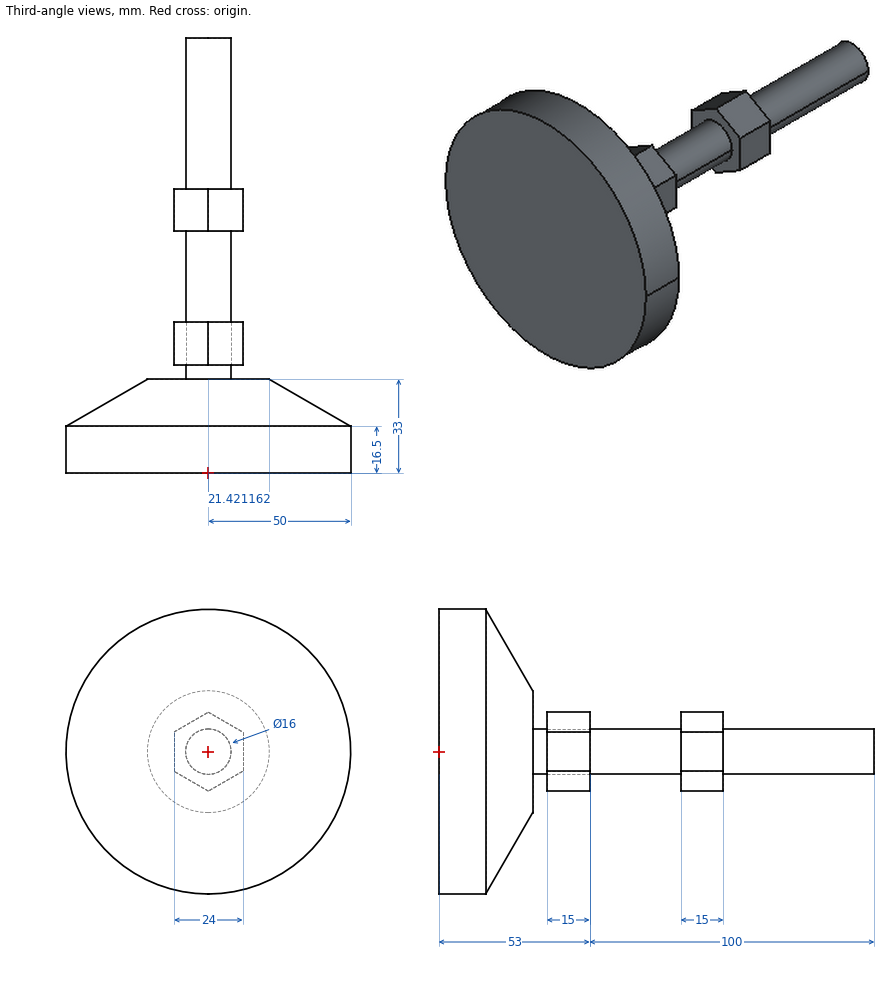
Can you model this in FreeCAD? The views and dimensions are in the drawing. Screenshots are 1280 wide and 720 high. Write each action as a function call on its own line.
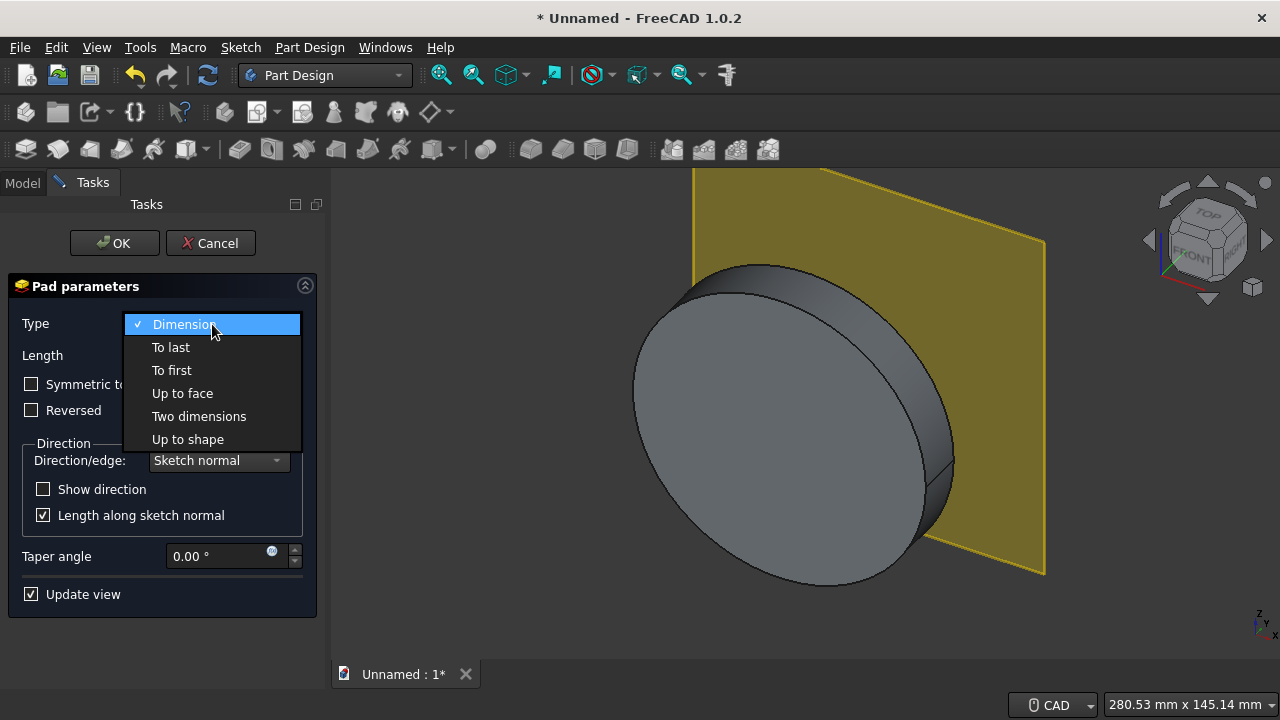
click(212, 416)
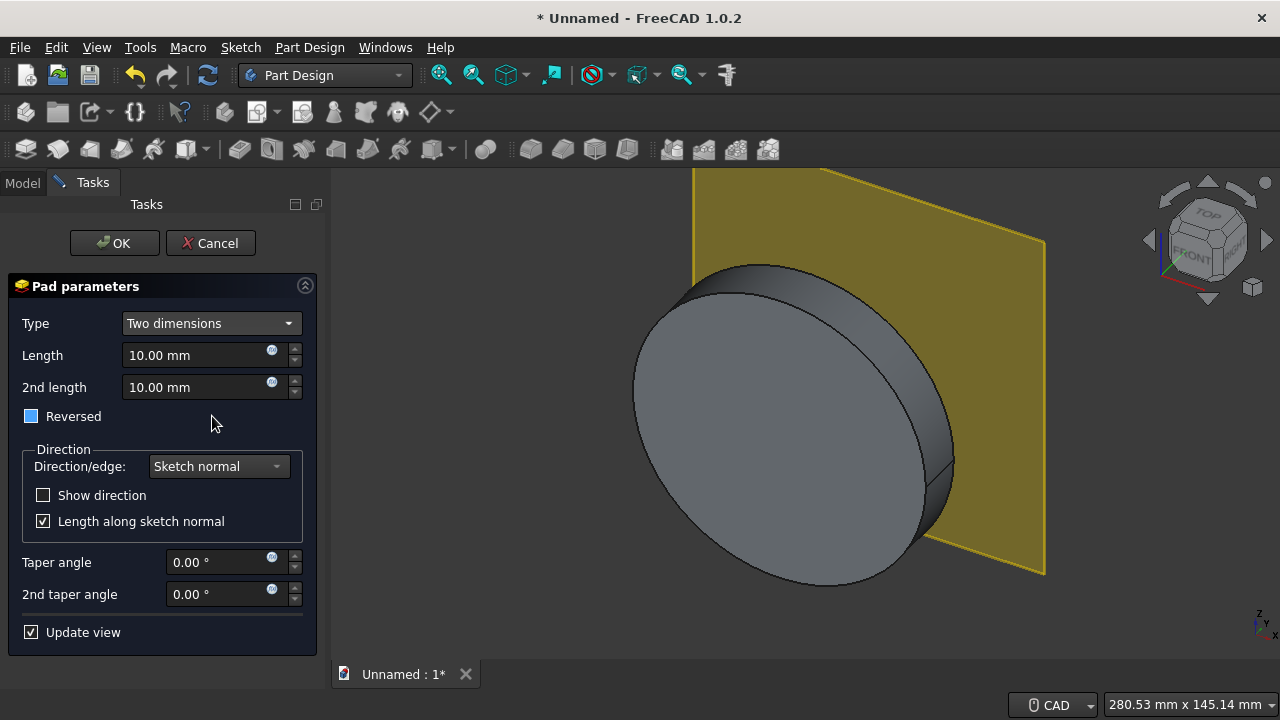
triple_click(204, 355)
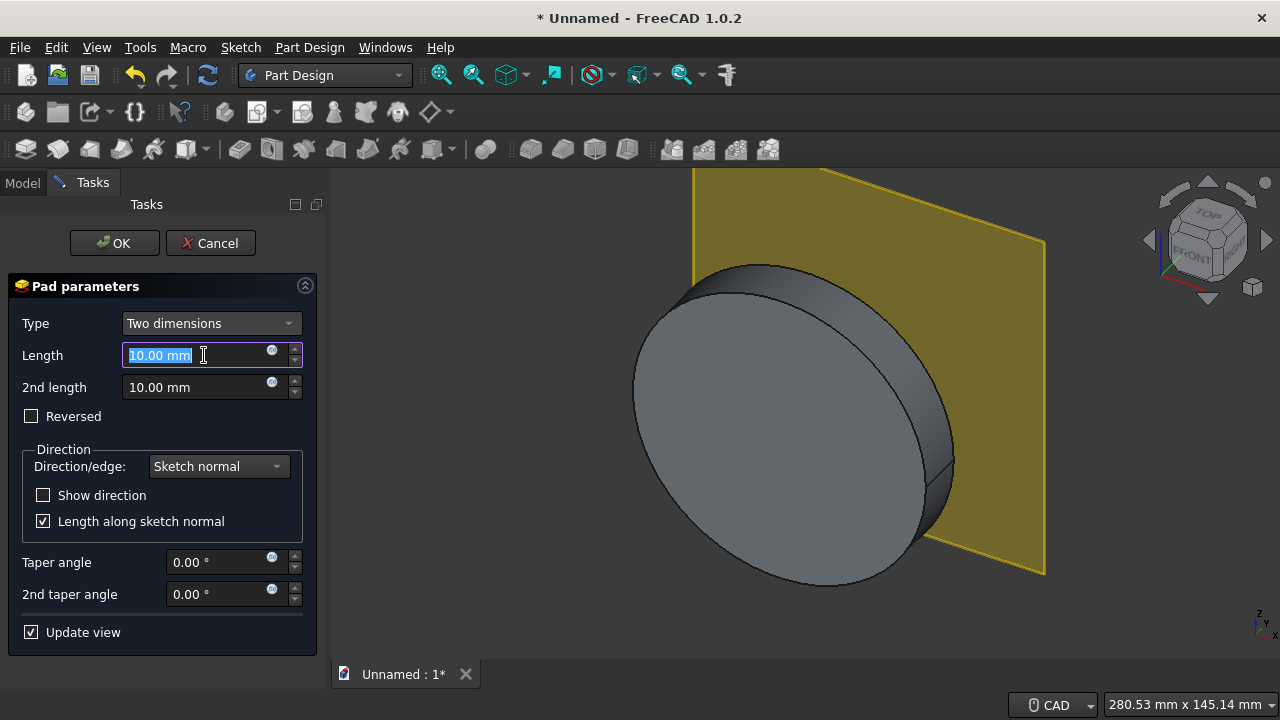
text(100)
key(Tab)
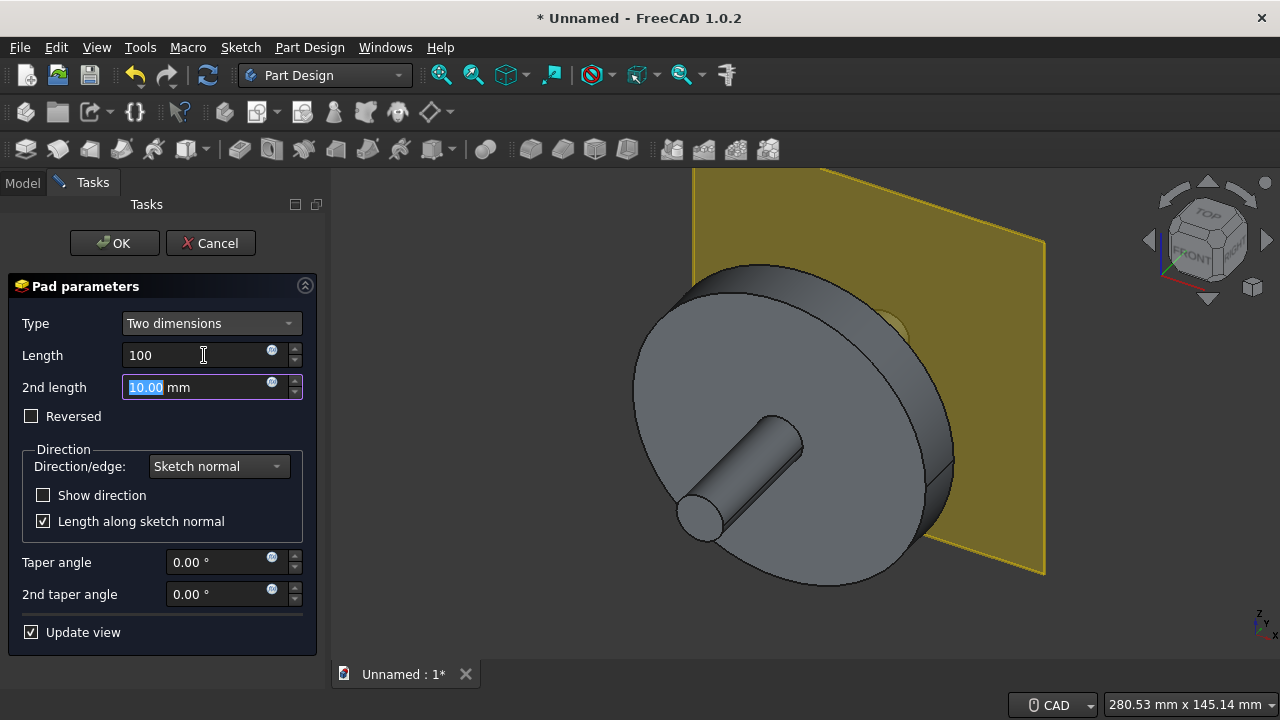
text(53)
key(Tab)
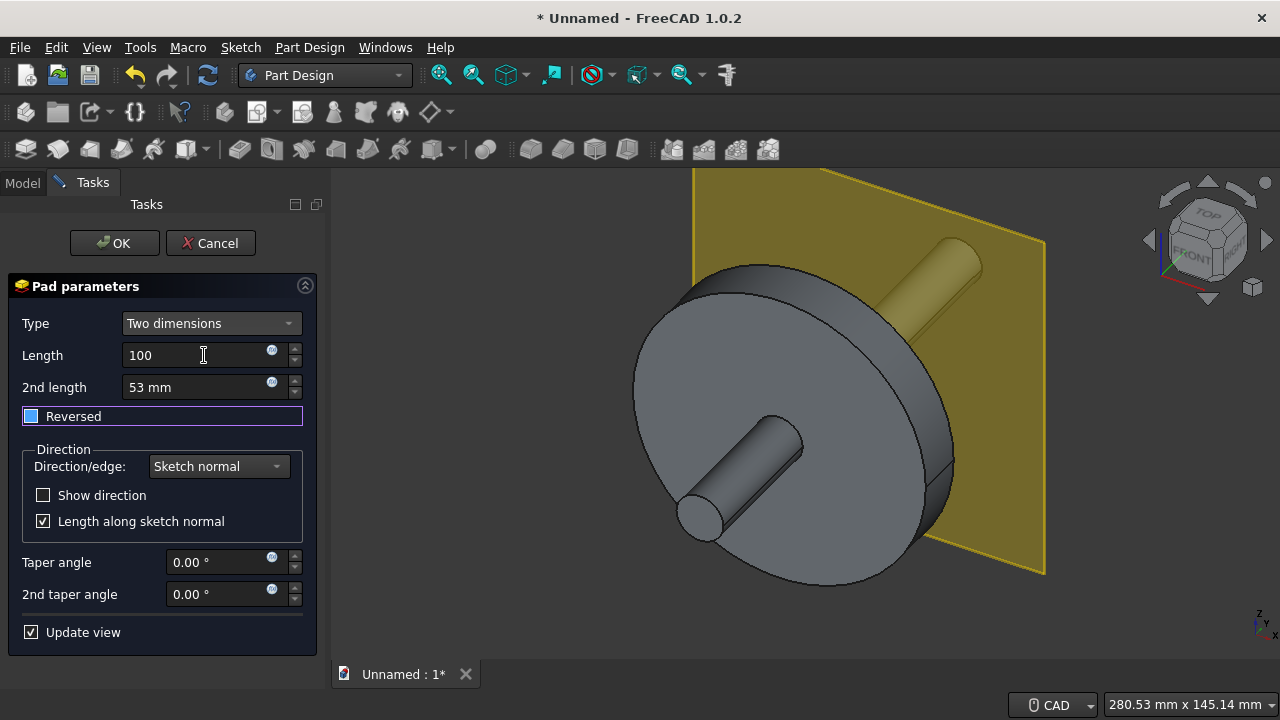
click(30, 416)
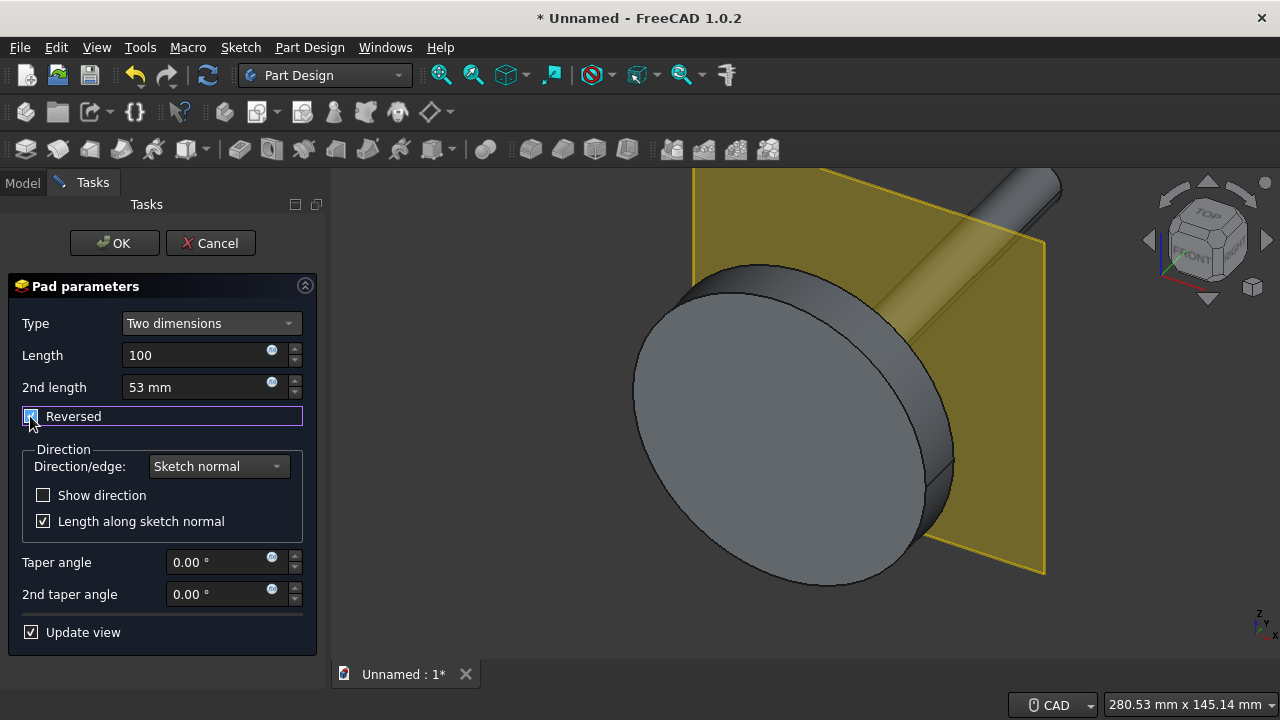
click(115, 243)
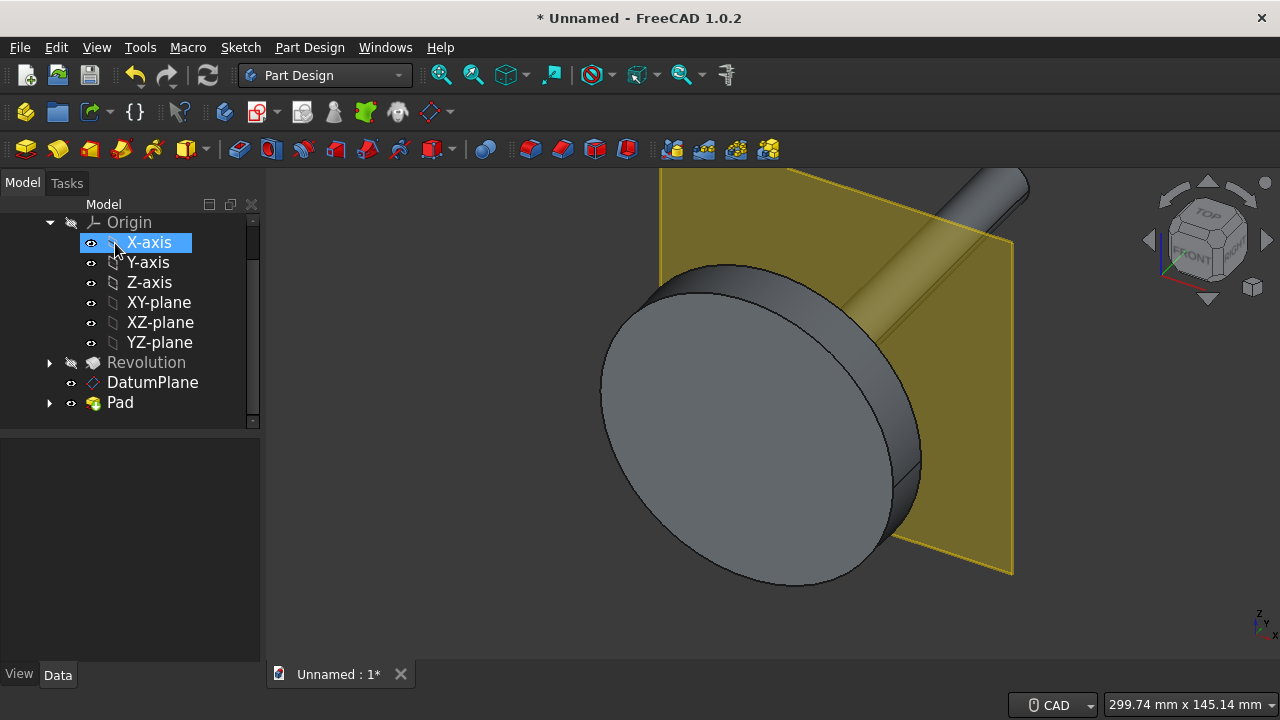
click(116, 383)
key(space)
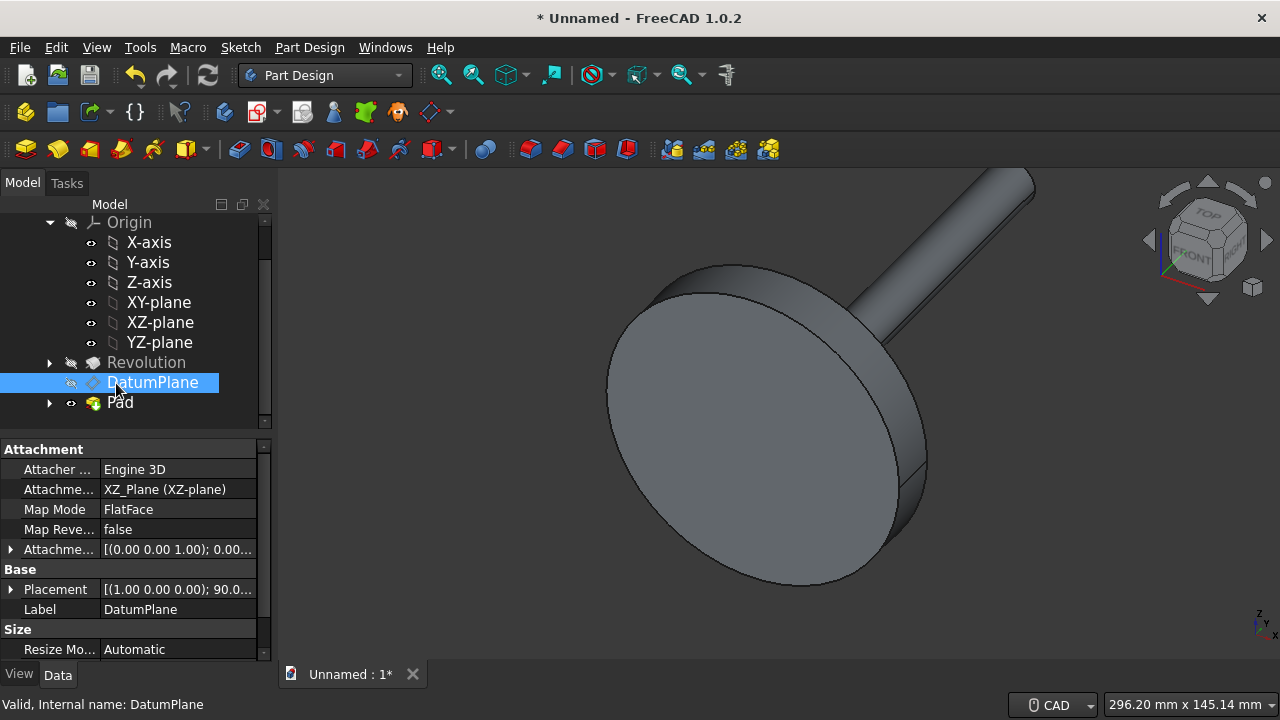
click(442, 76)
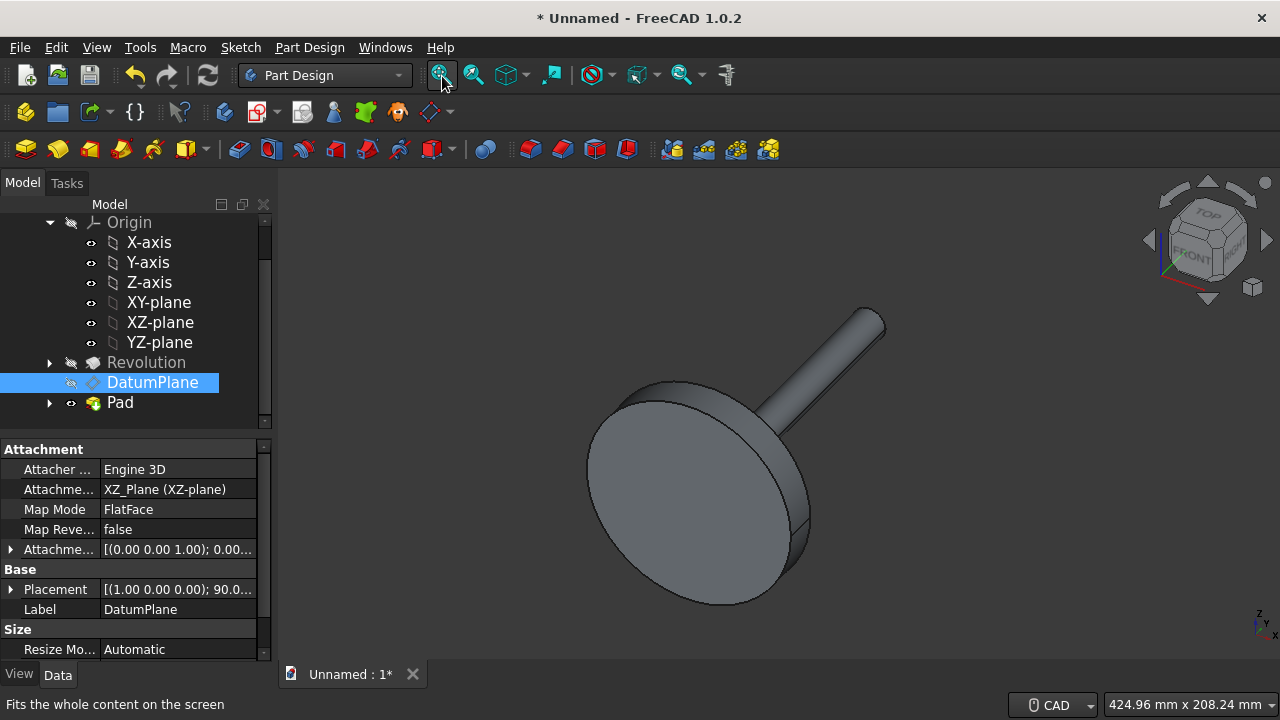
click(136, 323)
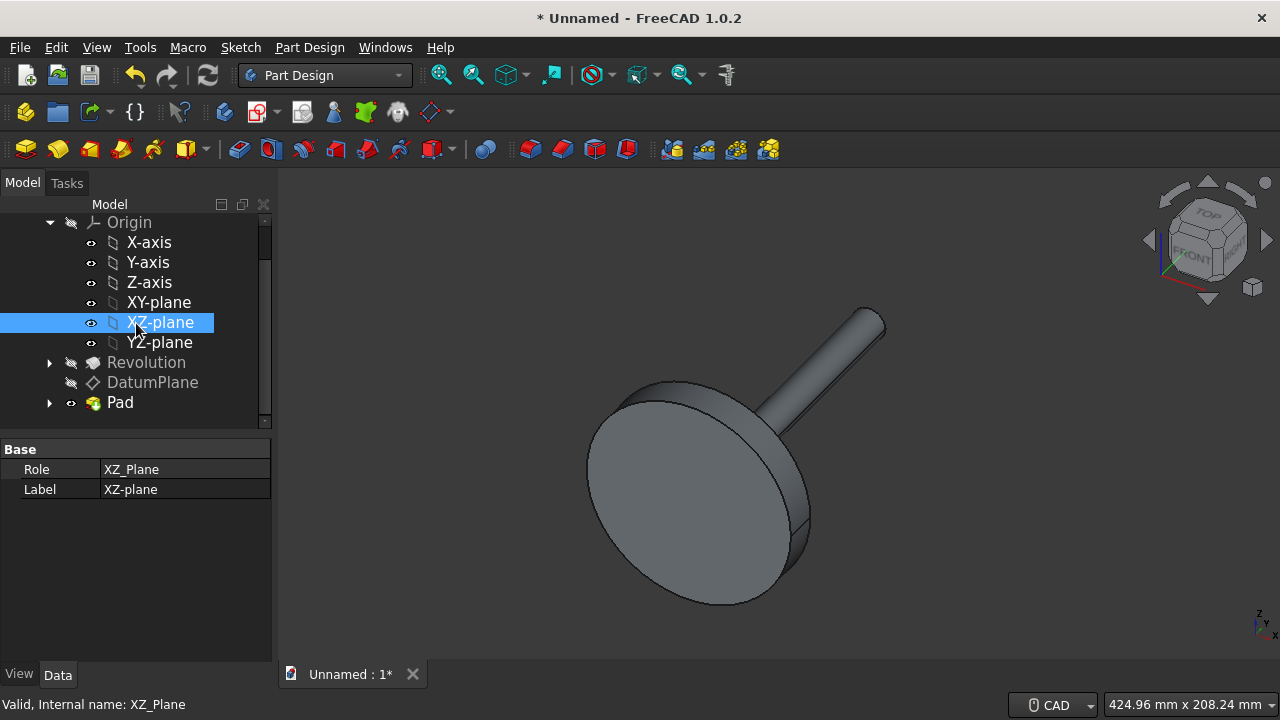
click(430, 112)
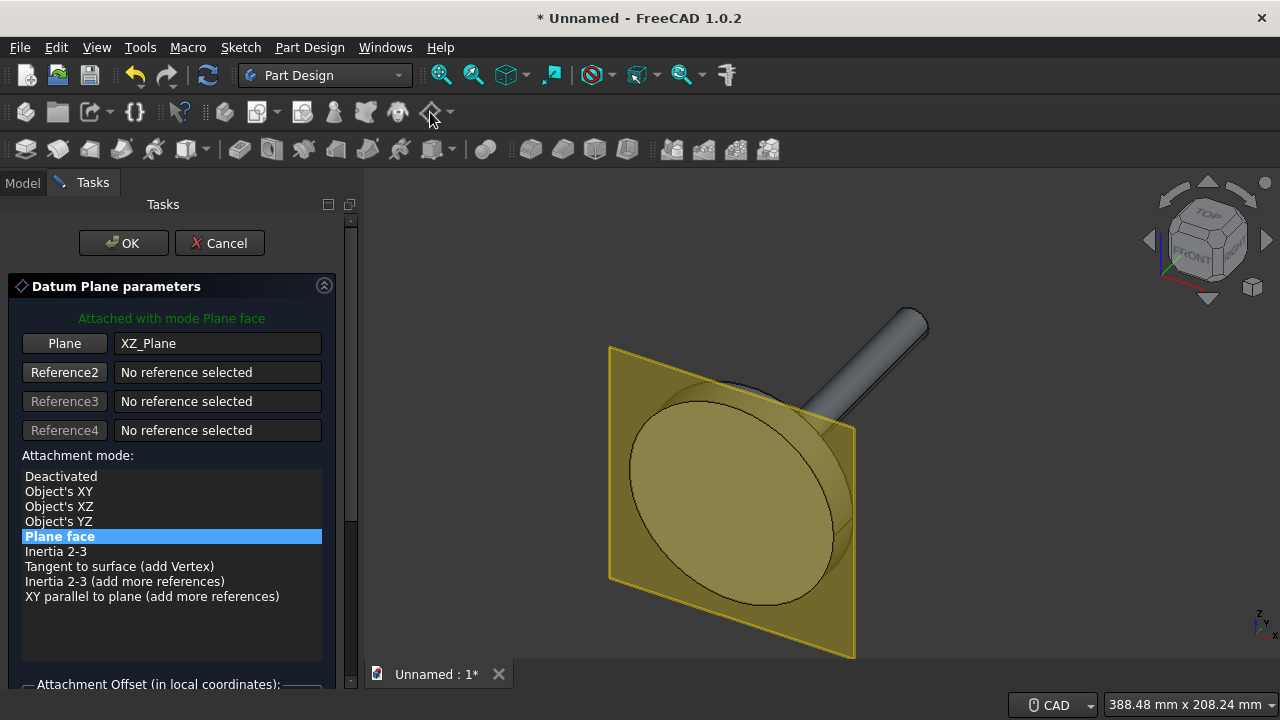
scroll(351, 451, down, 3)